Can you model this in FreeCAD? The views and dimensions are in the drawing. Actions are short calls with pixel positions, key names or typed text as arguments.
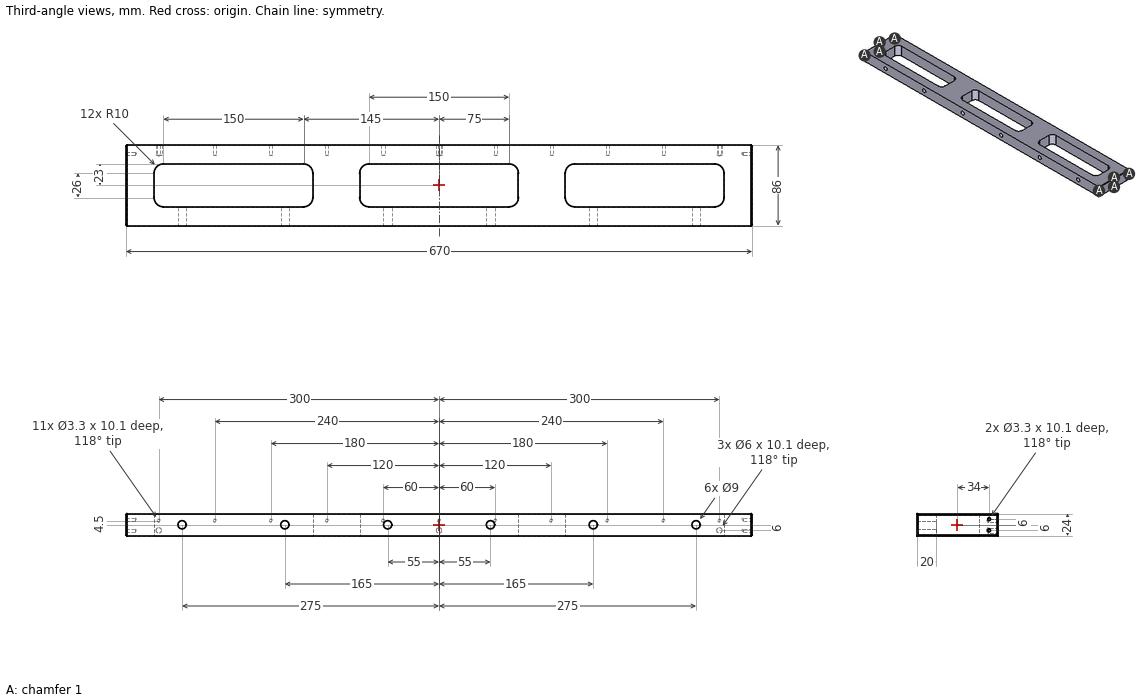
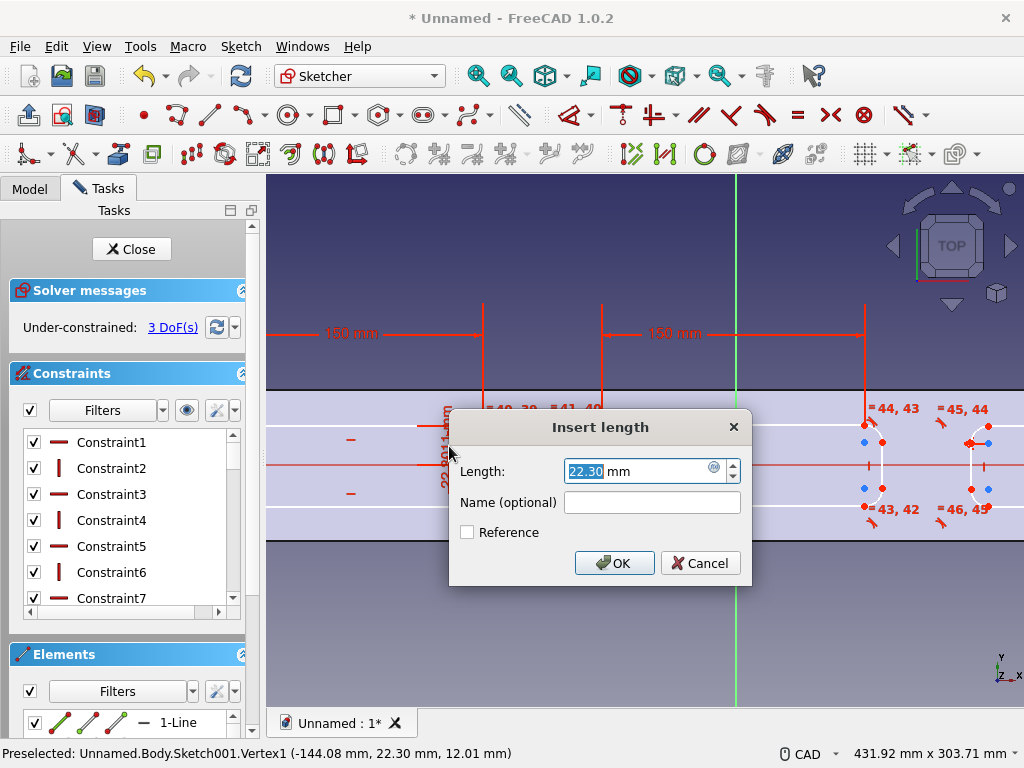
text(23)
key(Return)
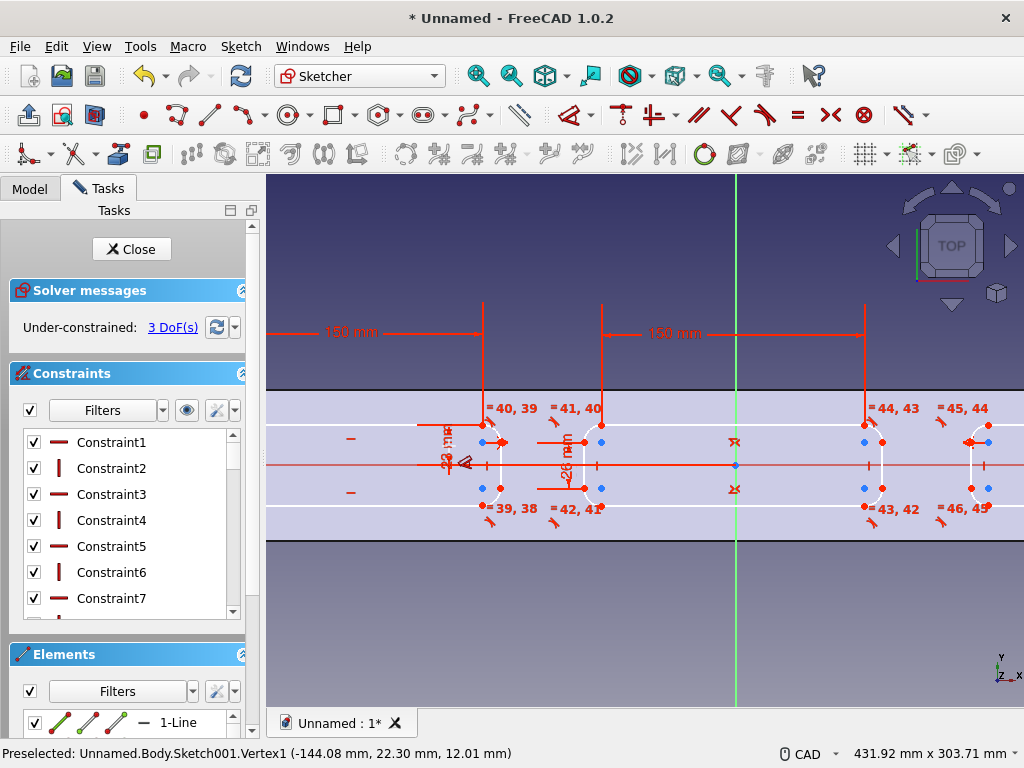
scroll(484, 426, down, 5)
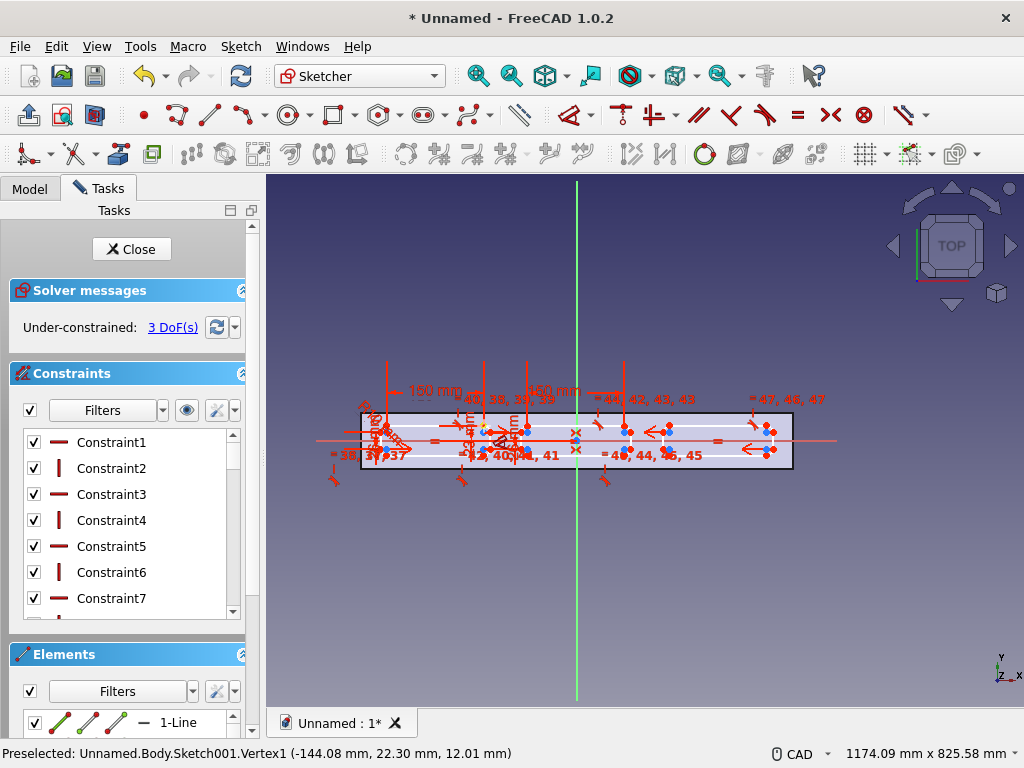
scroll(624, 426, up, 4)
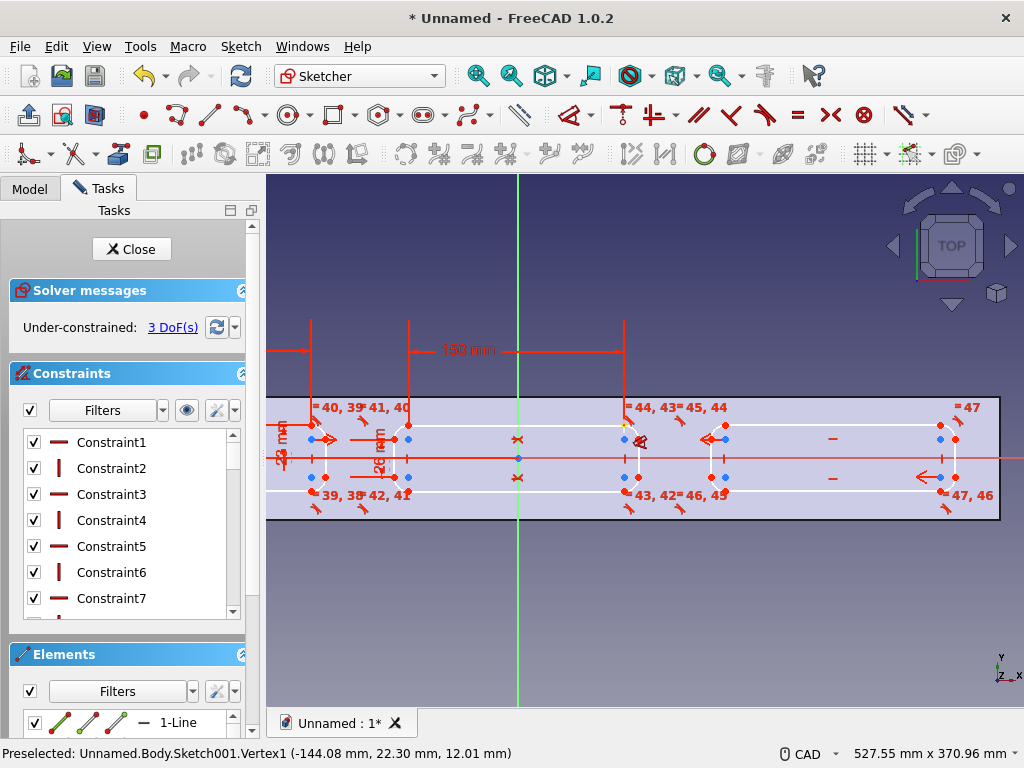
click(624, 426)
click(571, 392)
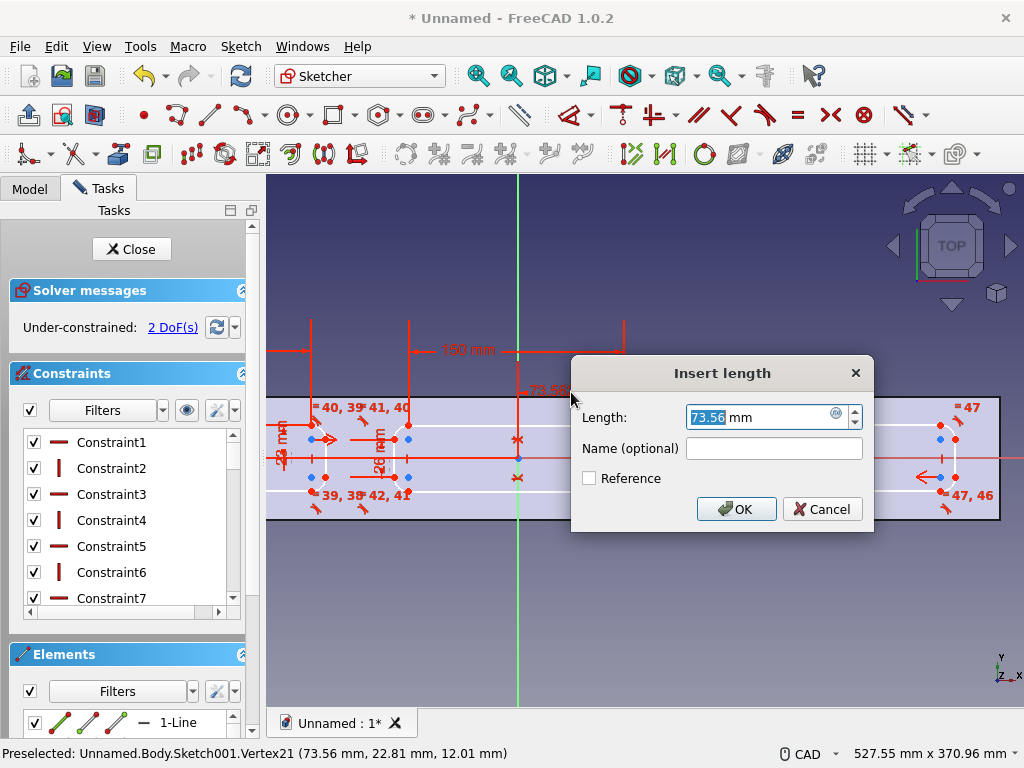
text(75)
key(Return)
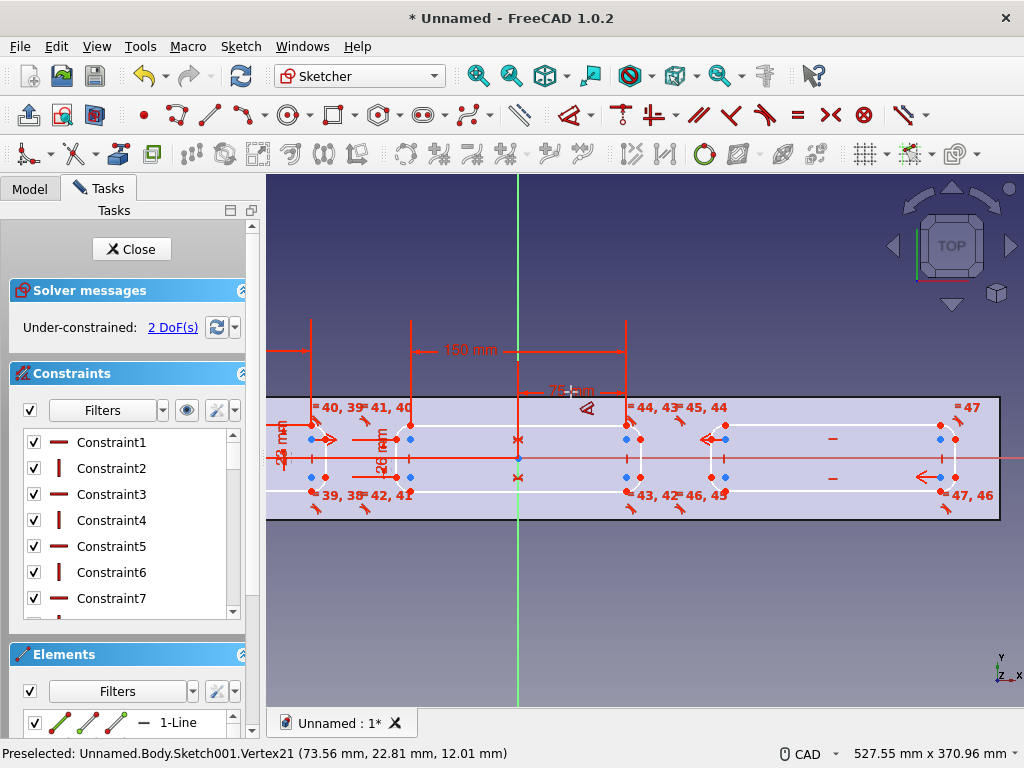
click(626, 426)
click(660, 442)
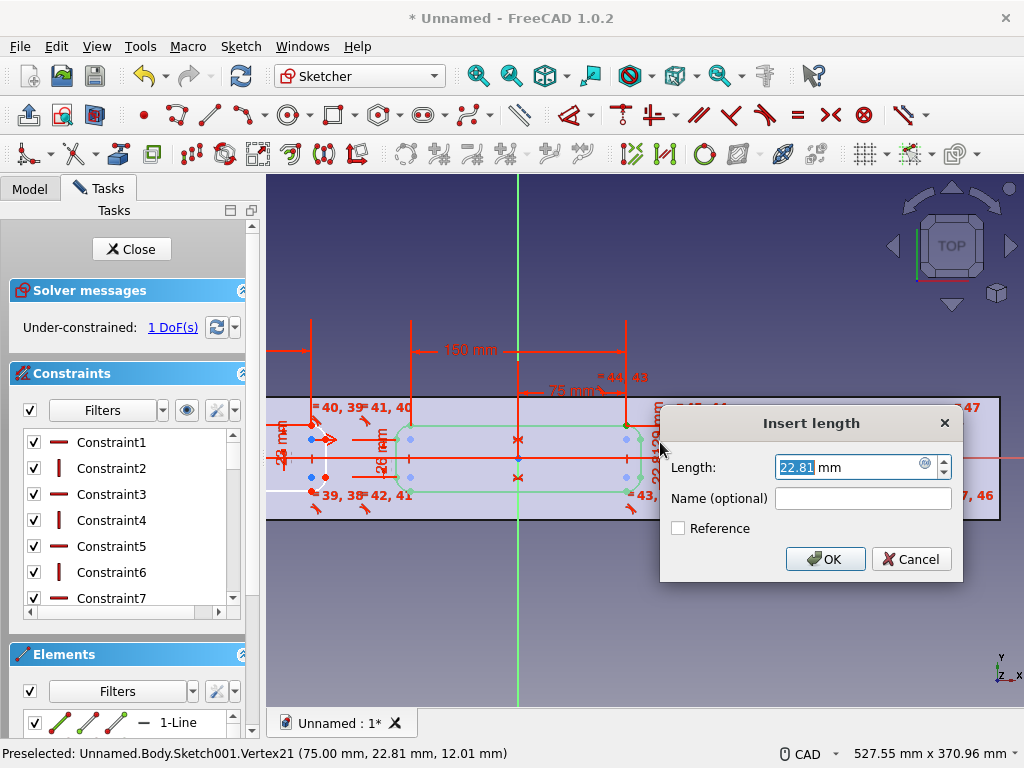
text(23)
key(Return)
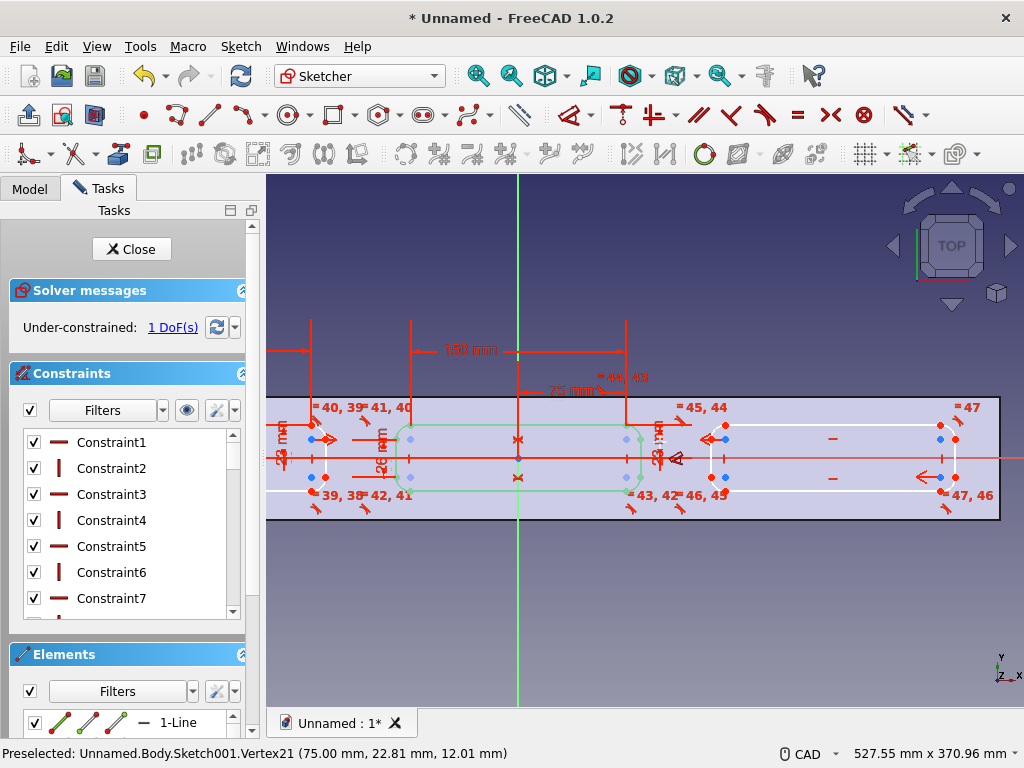
click(311, 425)
click(415, 391)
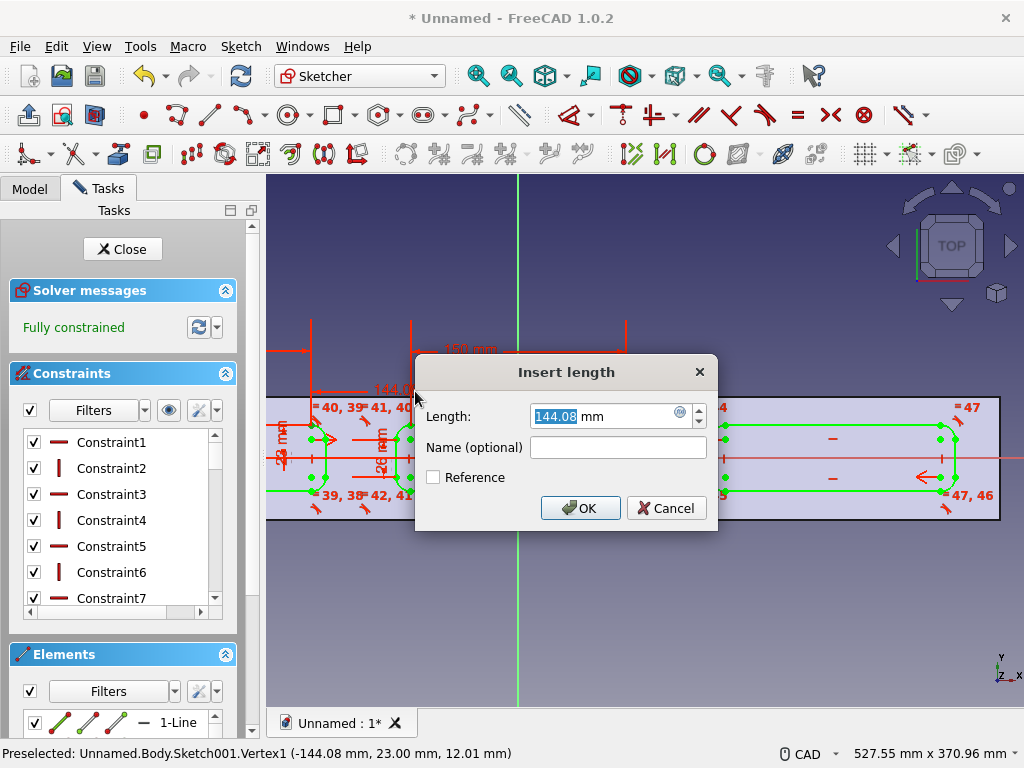
text(145)
key(Return)
key(Escape)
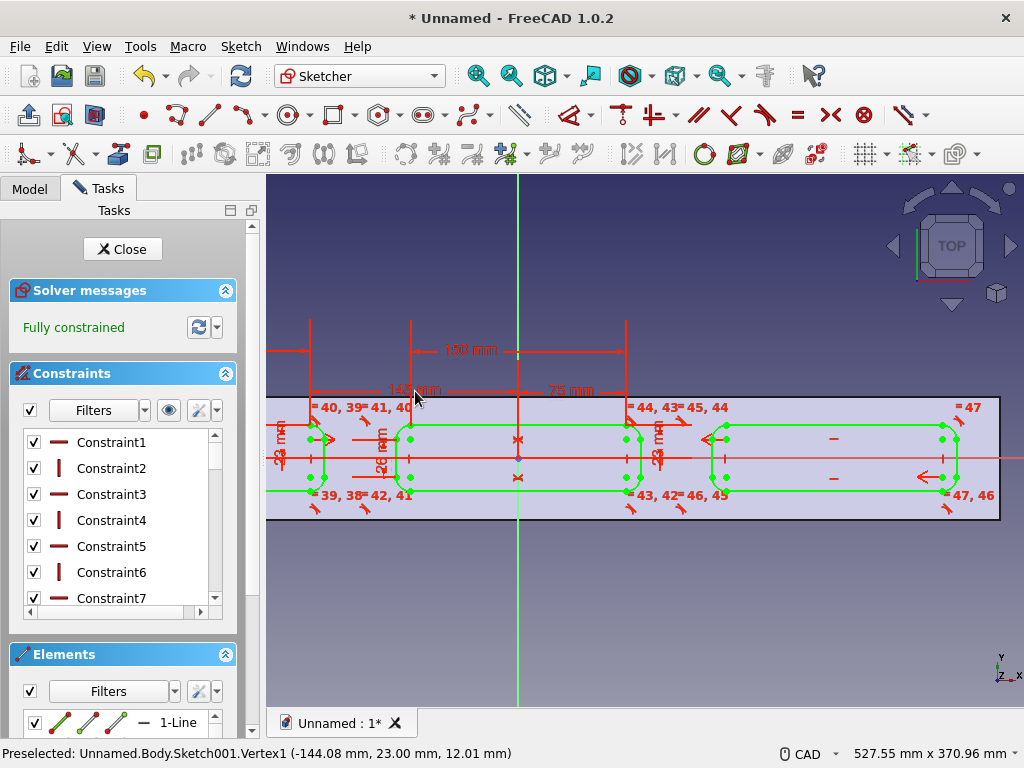
click(123, 249)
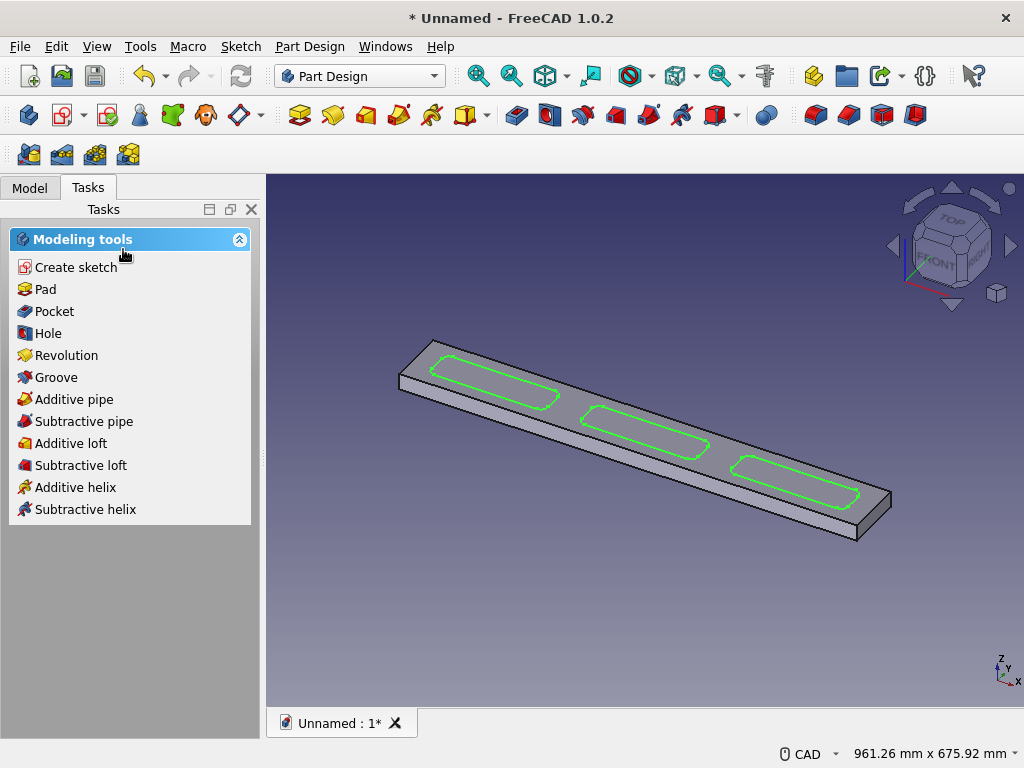
click(517, 116)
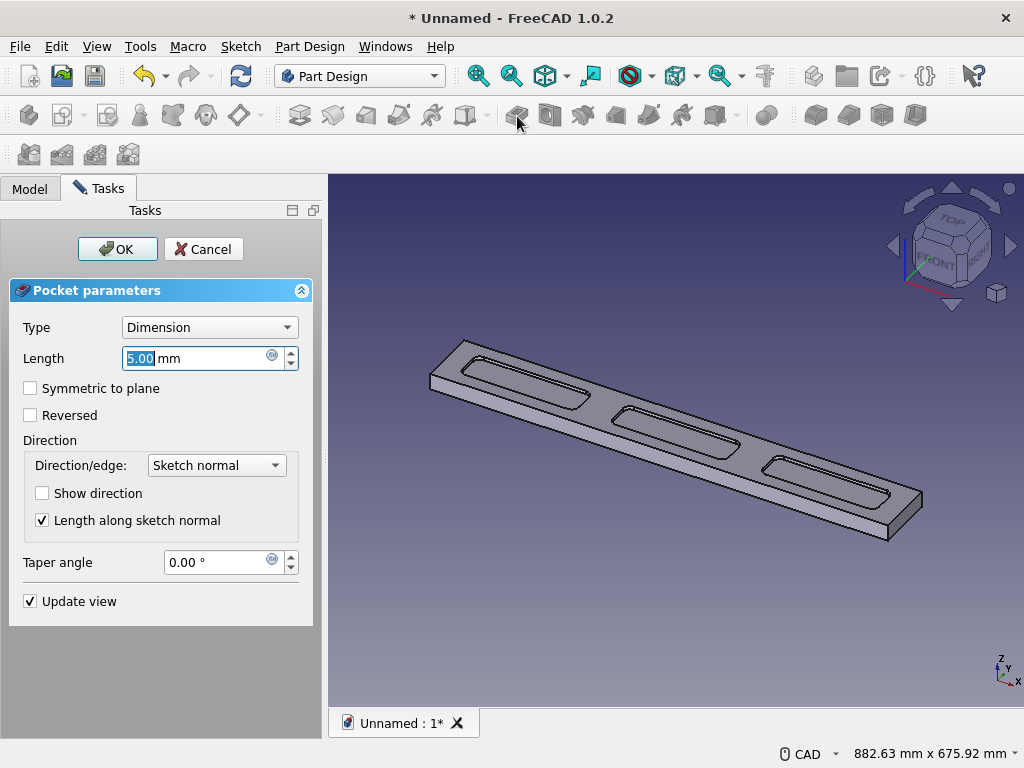
click(210, 328)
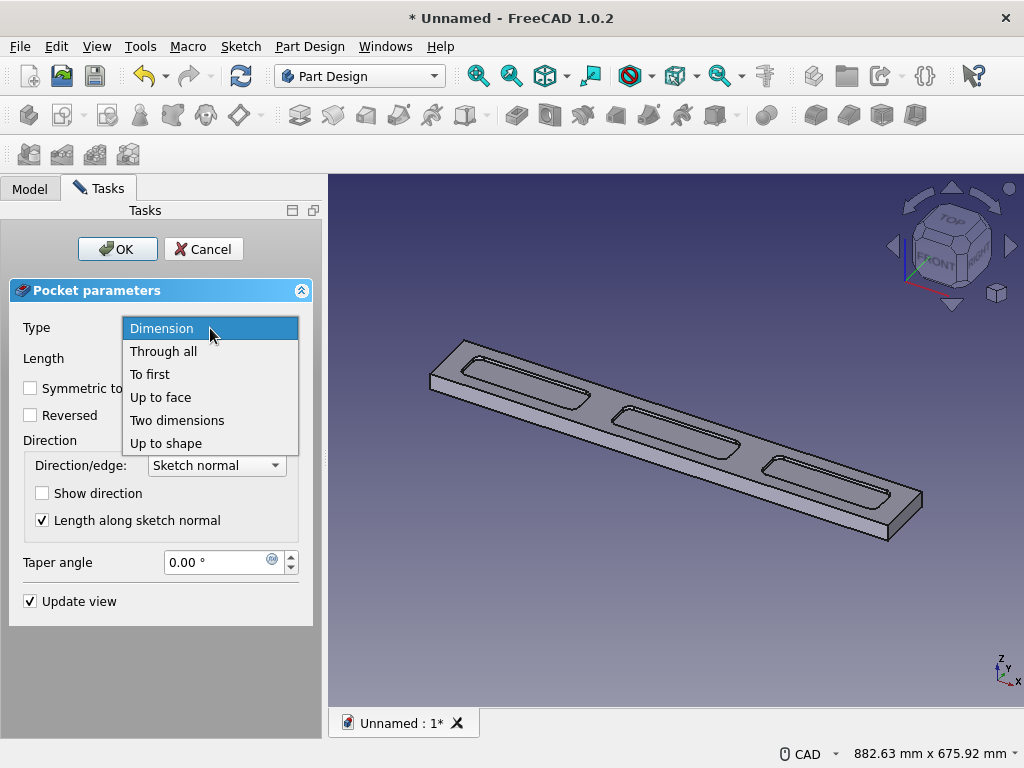
click(208, 352)